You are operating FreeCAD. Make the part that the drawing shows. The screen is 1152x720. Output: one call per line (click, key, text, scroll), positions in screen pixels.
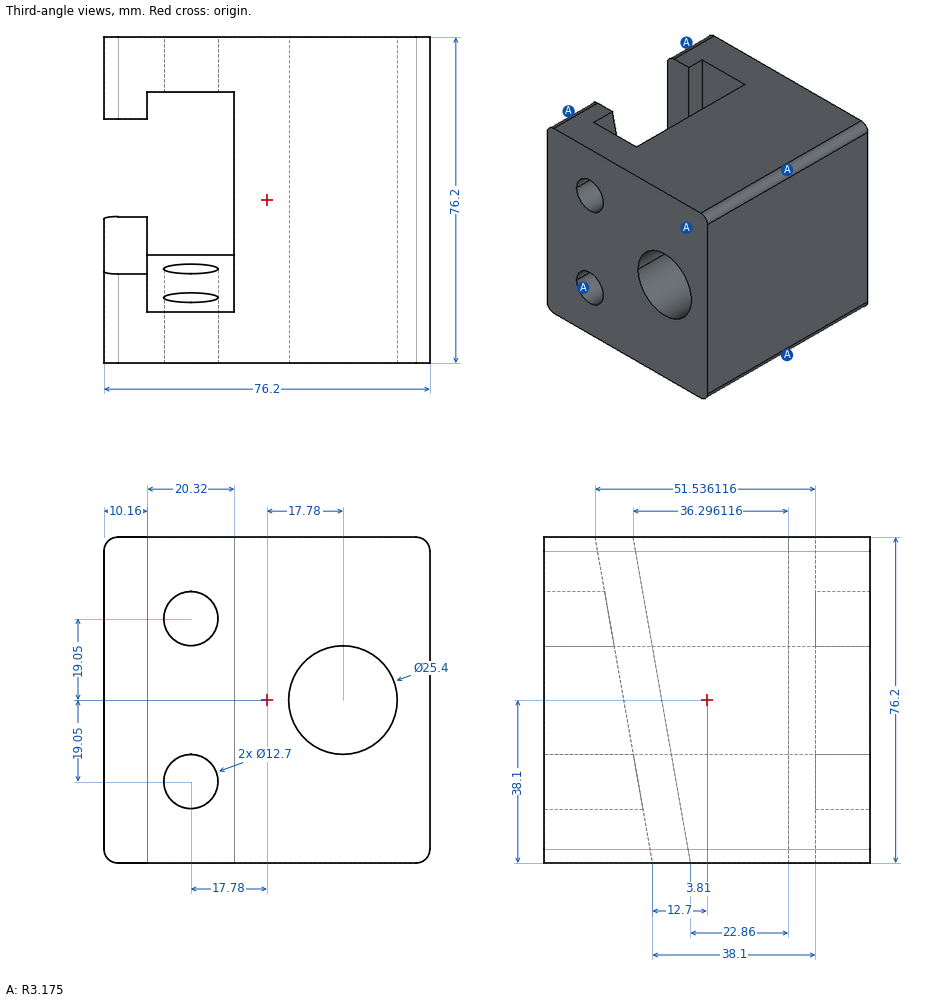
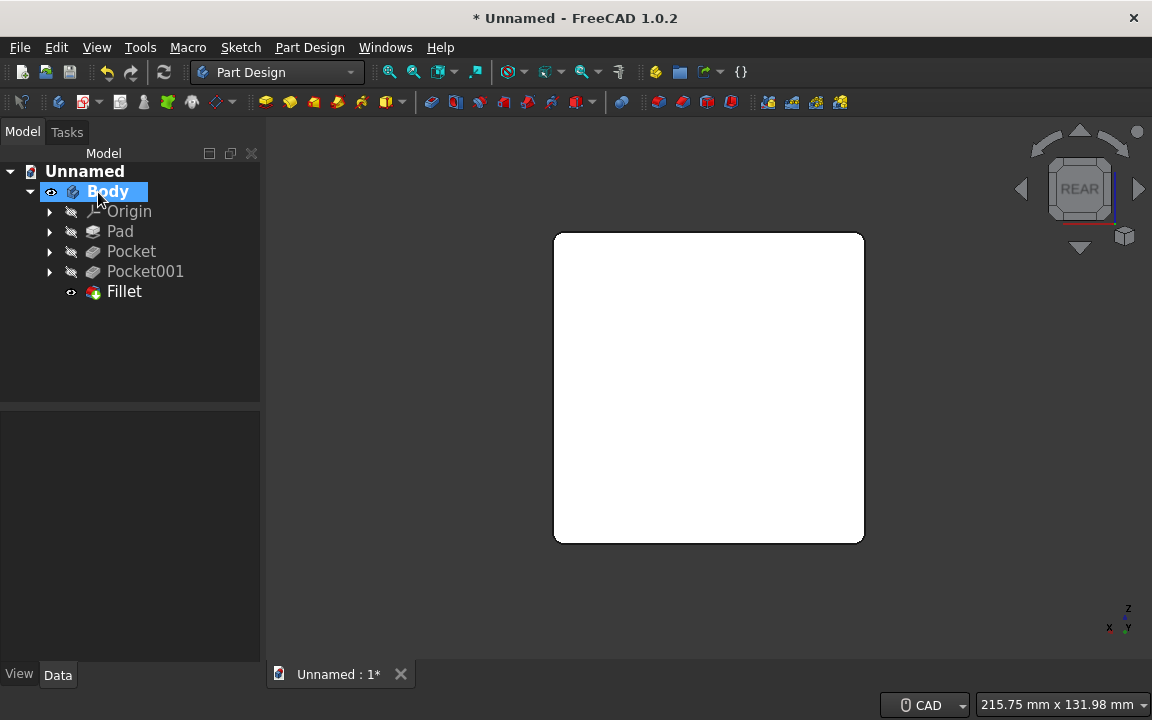
click(709, 387)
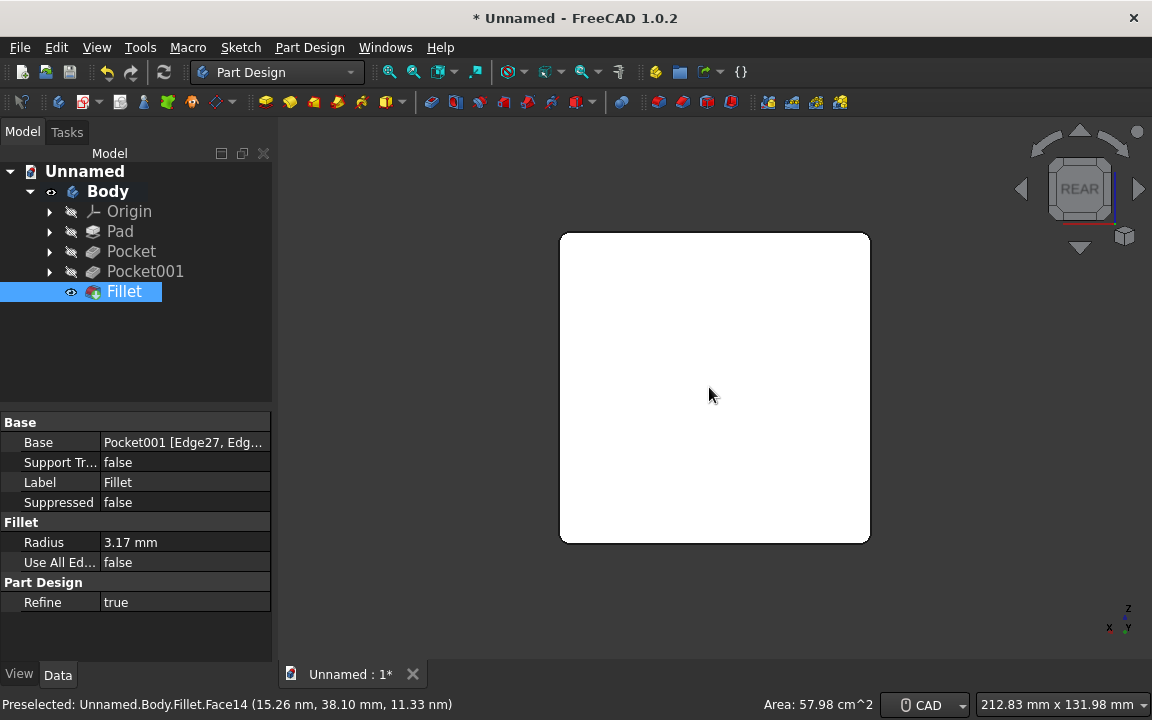
click(84, 102)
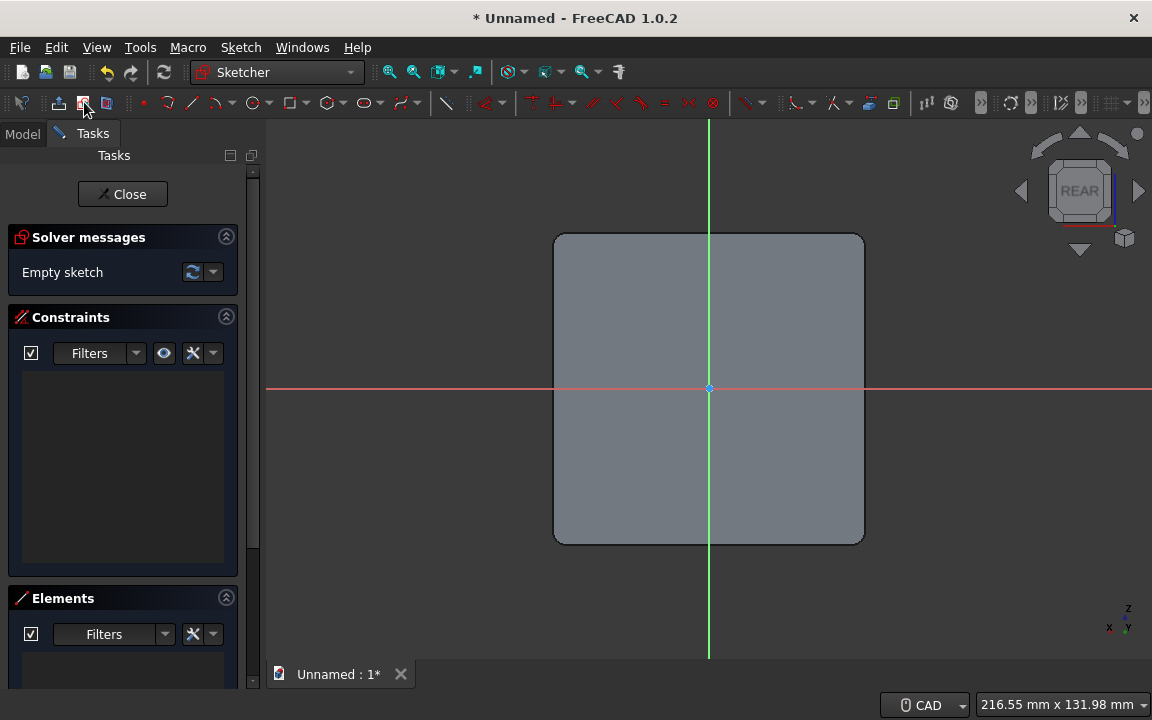
scroll(809, 389, up, 2)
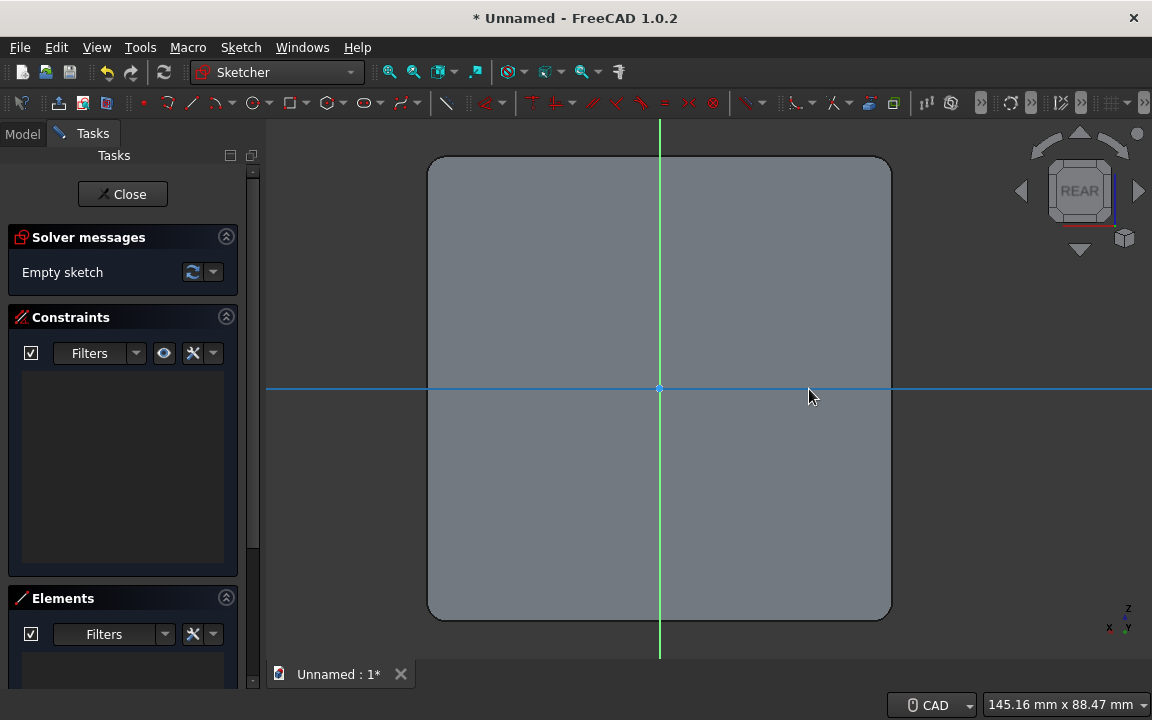
key(g)
key(c)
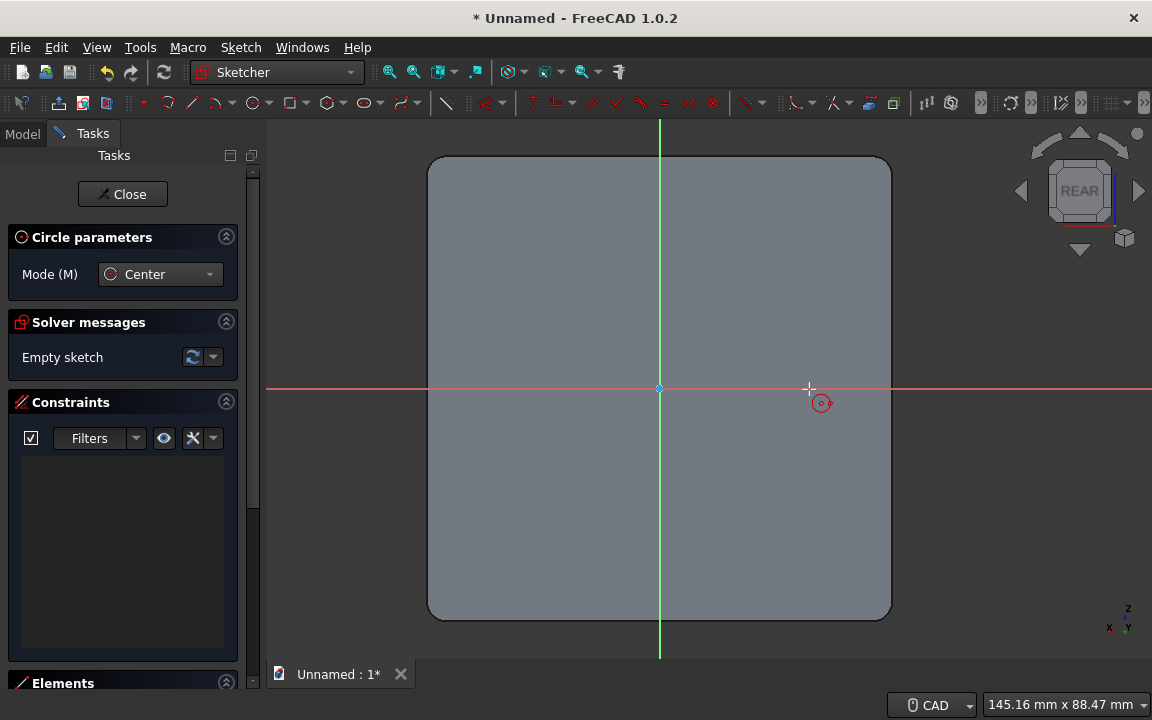
click(768, 505)
click(795, 478)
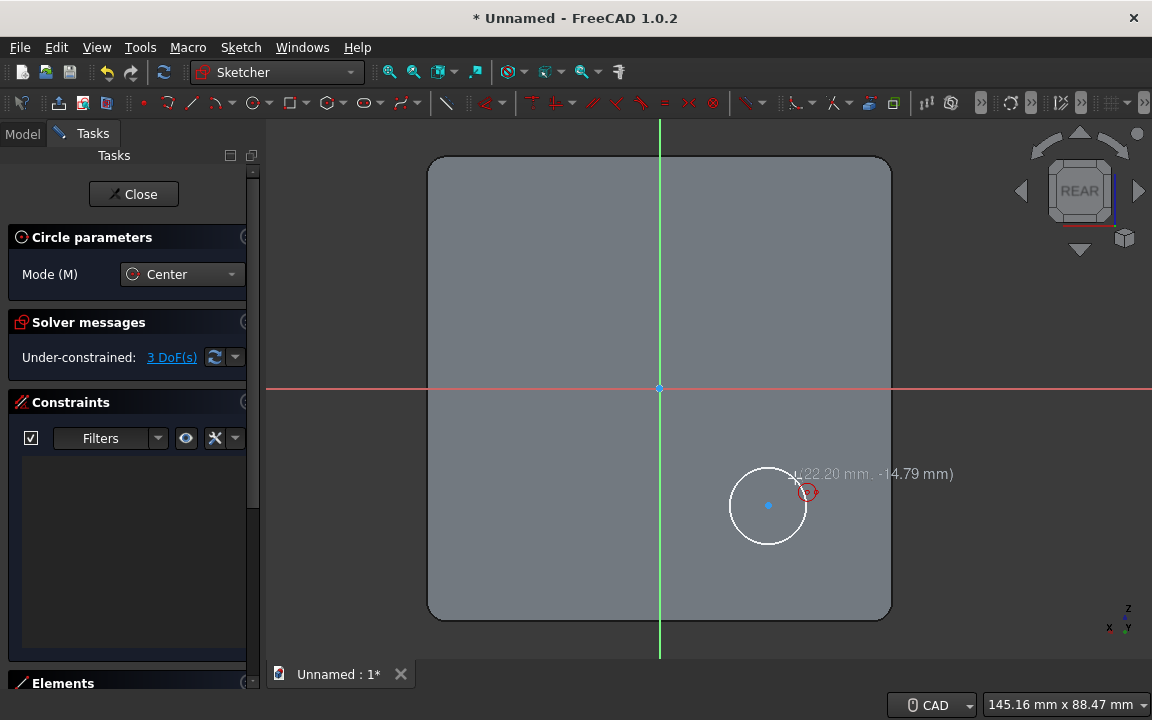
click(768, 272)
click(795, 245)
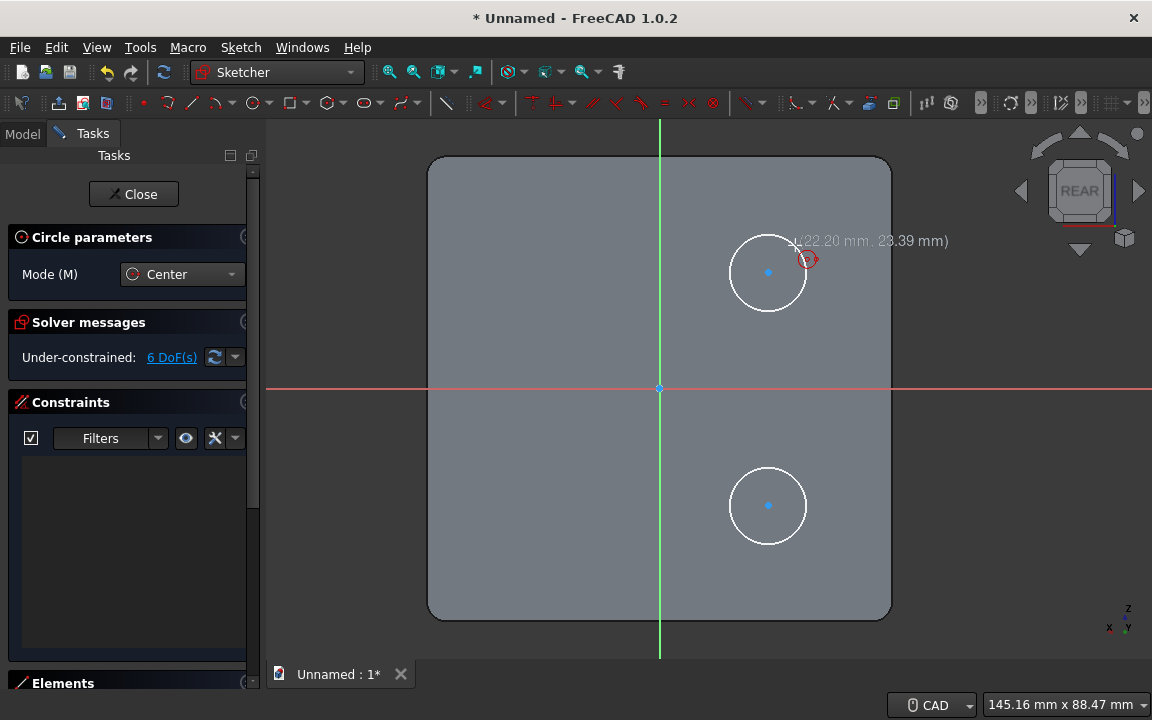
click(551, 389)
click(606, 334)
key(Escape)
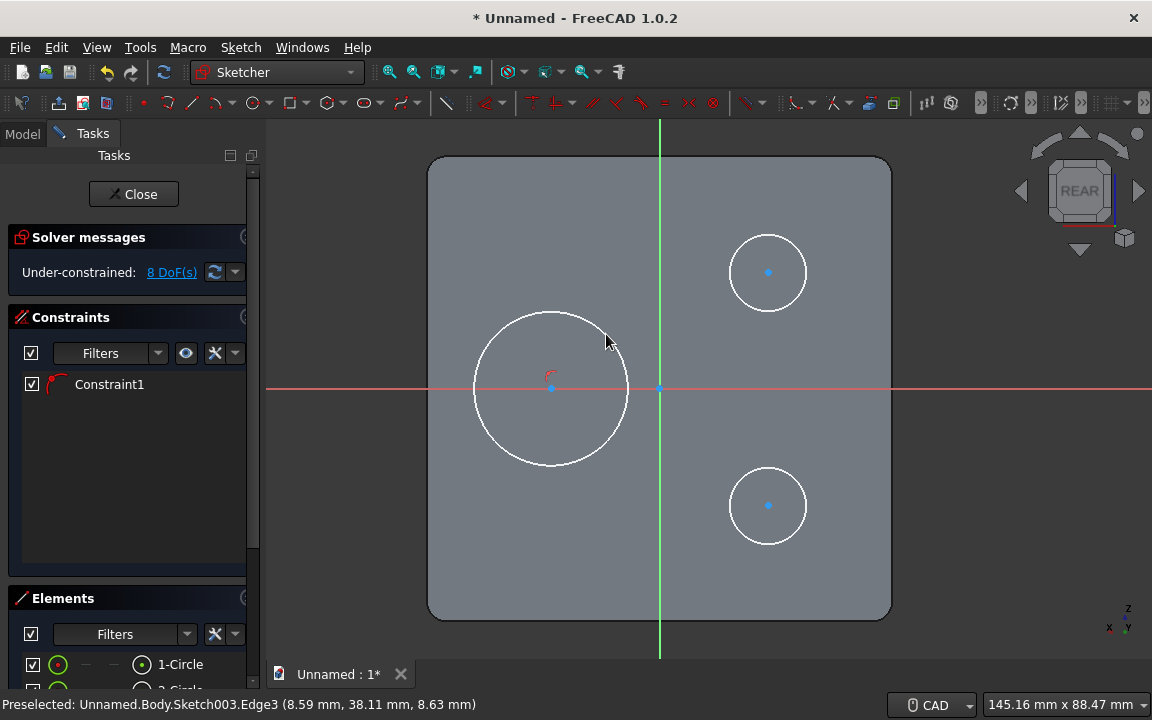
click(795, 479)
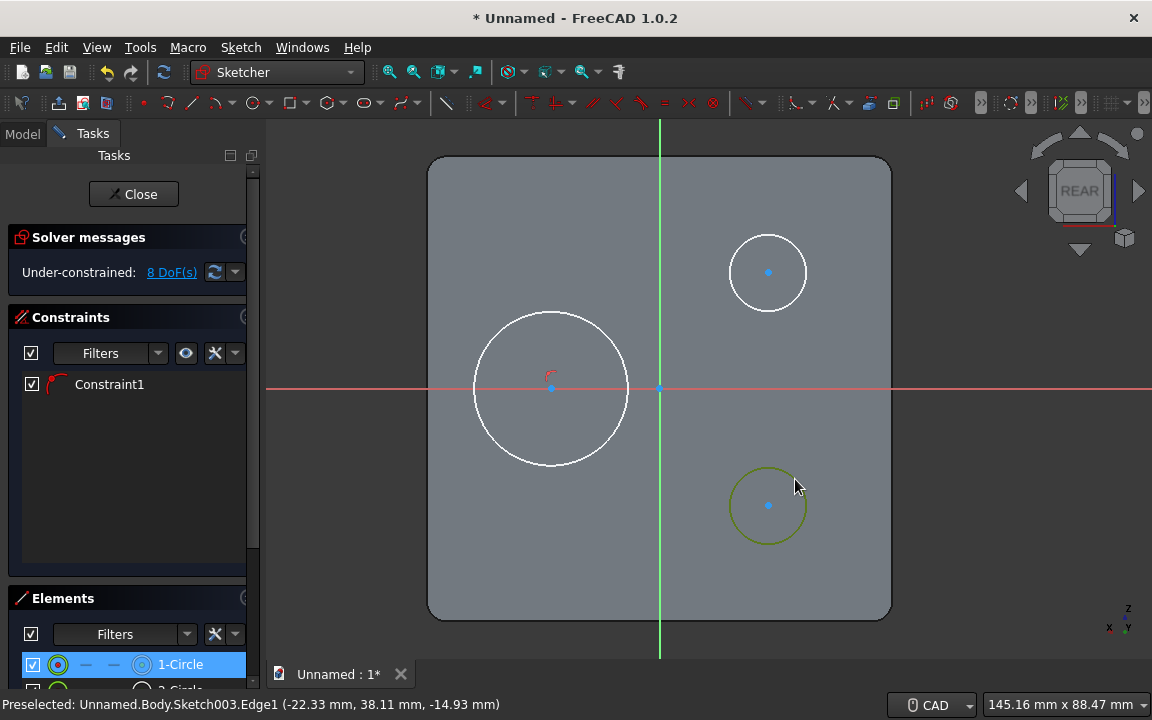
click(795, 246)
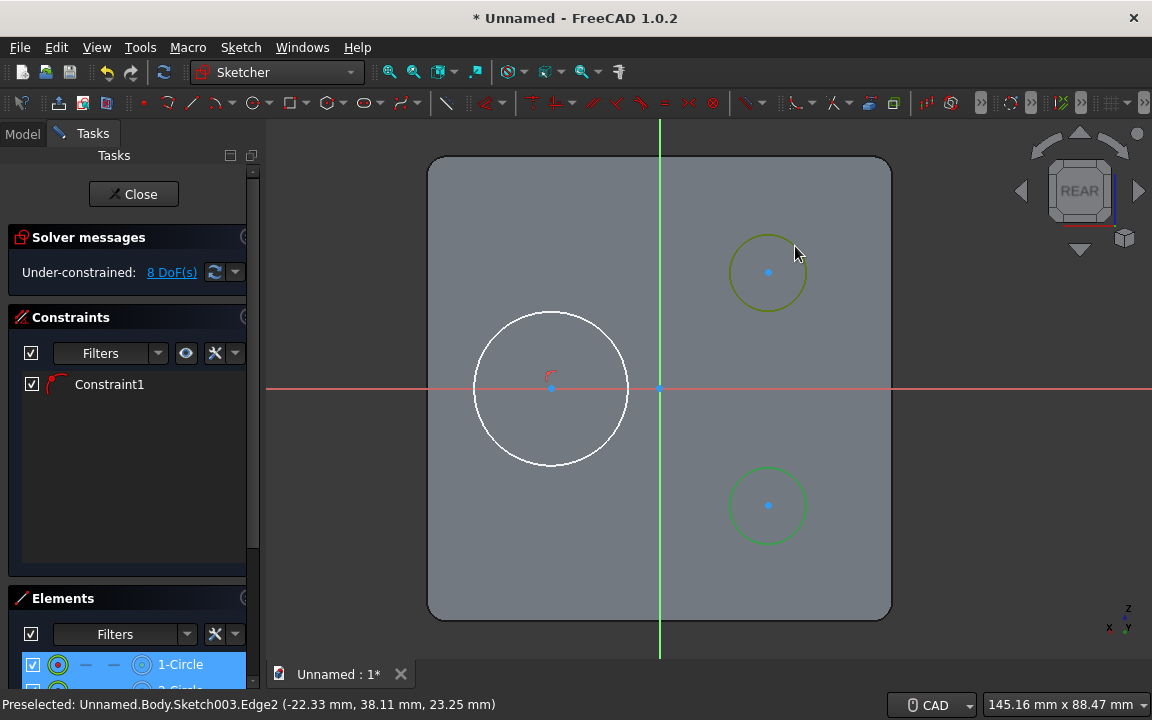
click(666, 104)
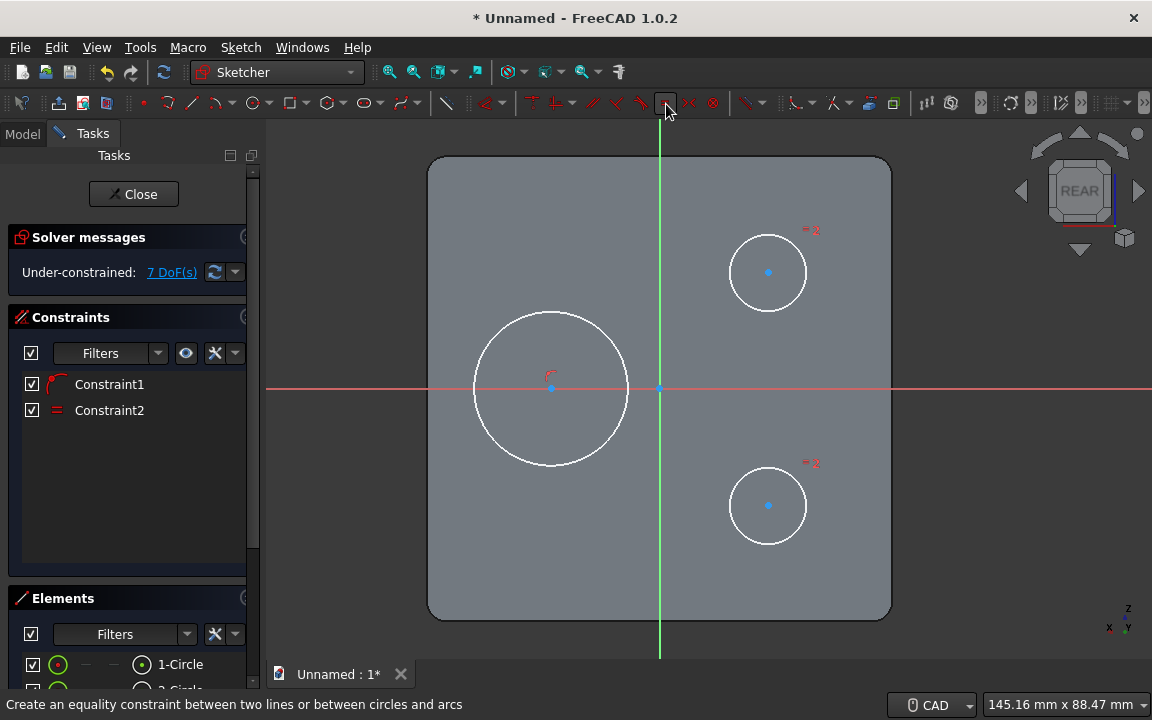
click(768, 506)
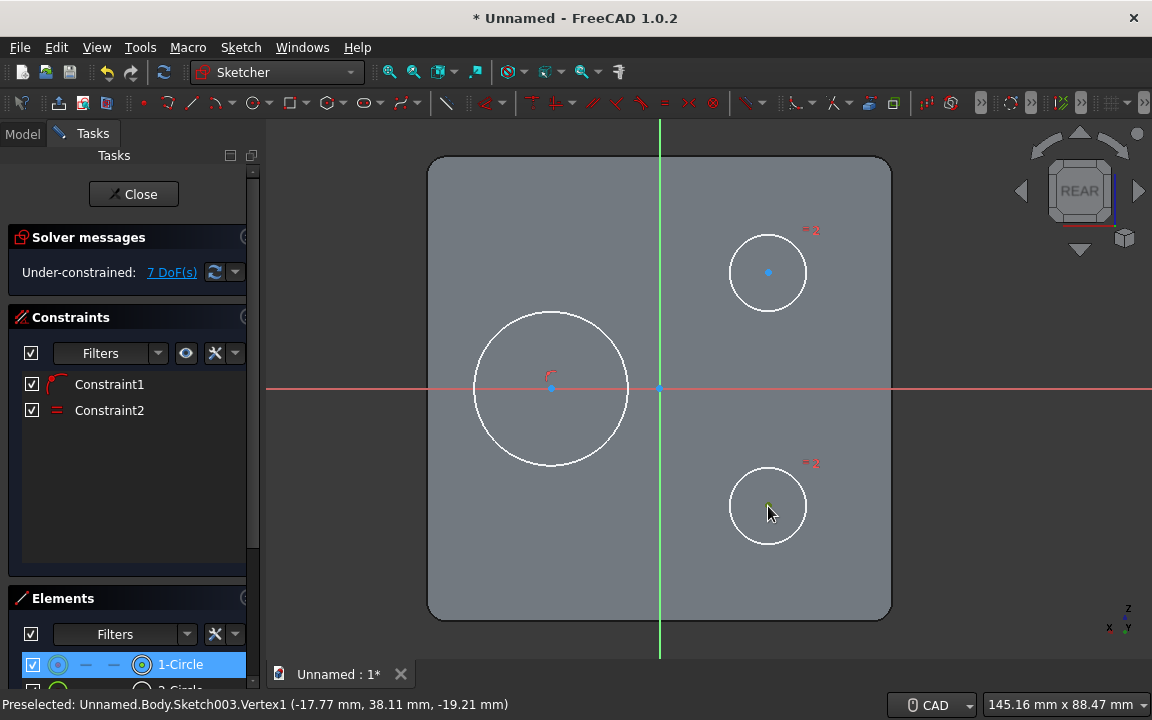
click(768, 273)